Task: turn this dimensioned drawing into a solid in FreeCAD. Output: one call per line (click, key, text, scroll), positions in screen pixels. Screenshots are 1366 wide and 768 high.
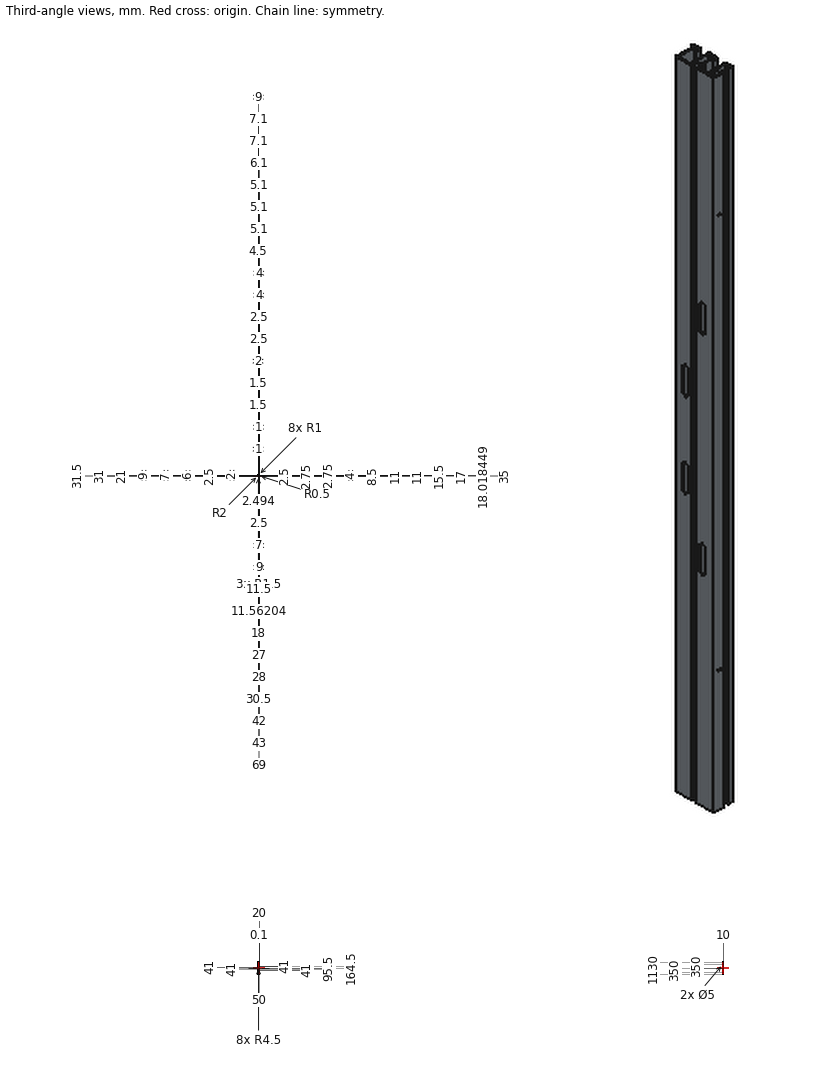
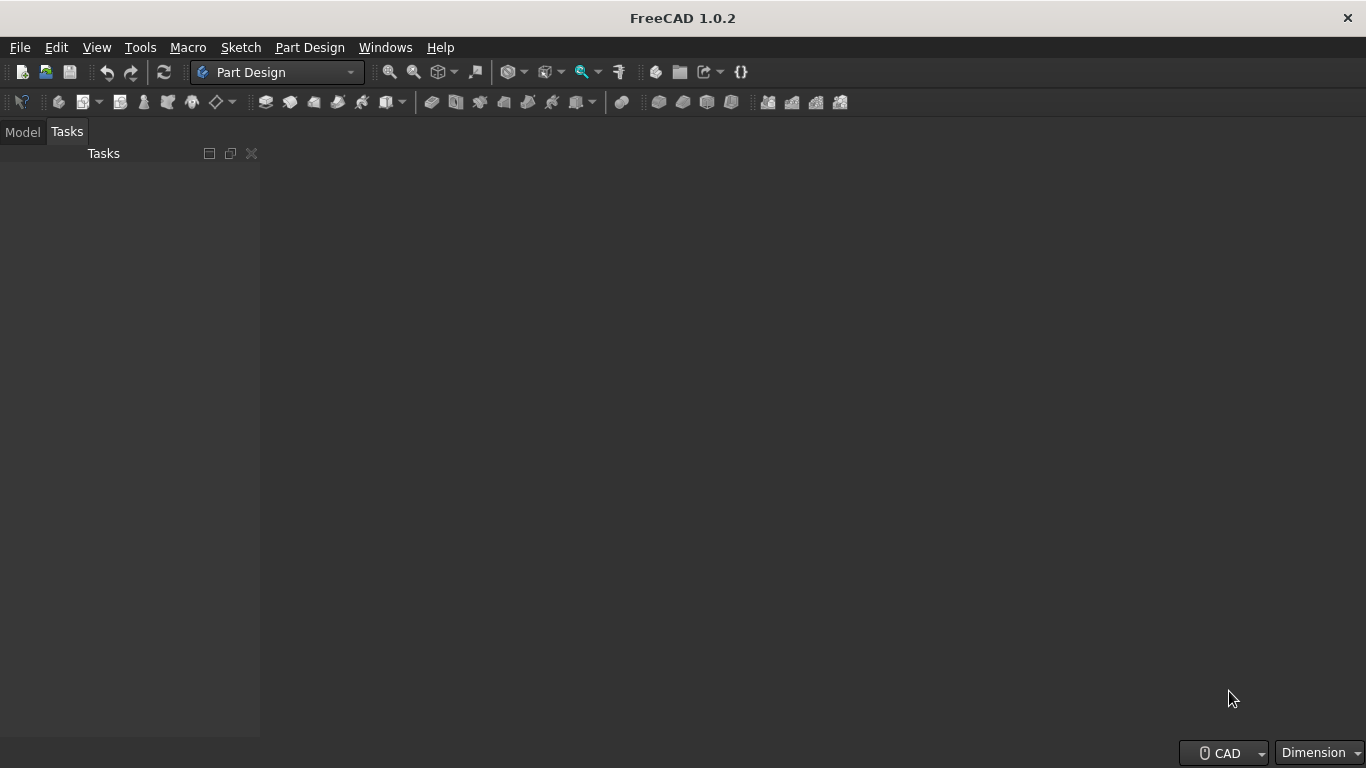
click(22, 72)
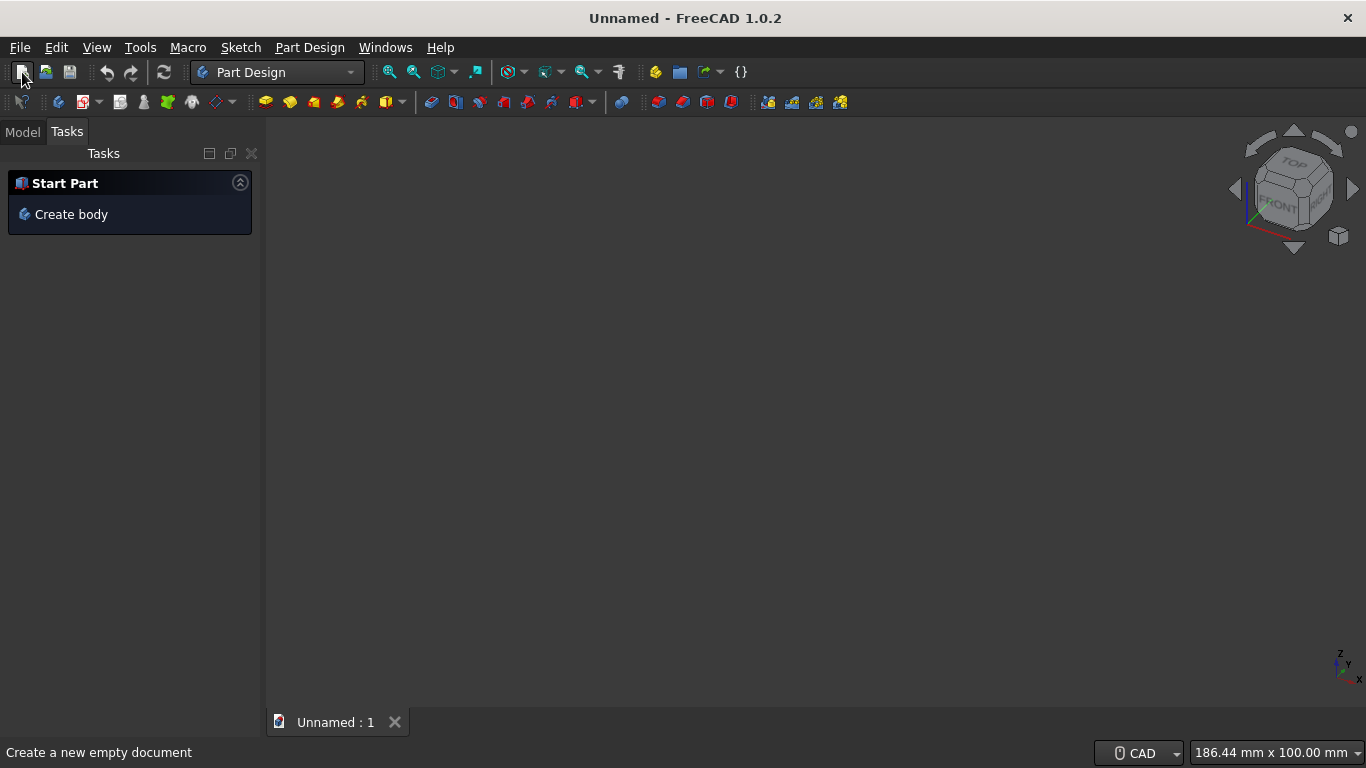
click(84, 102)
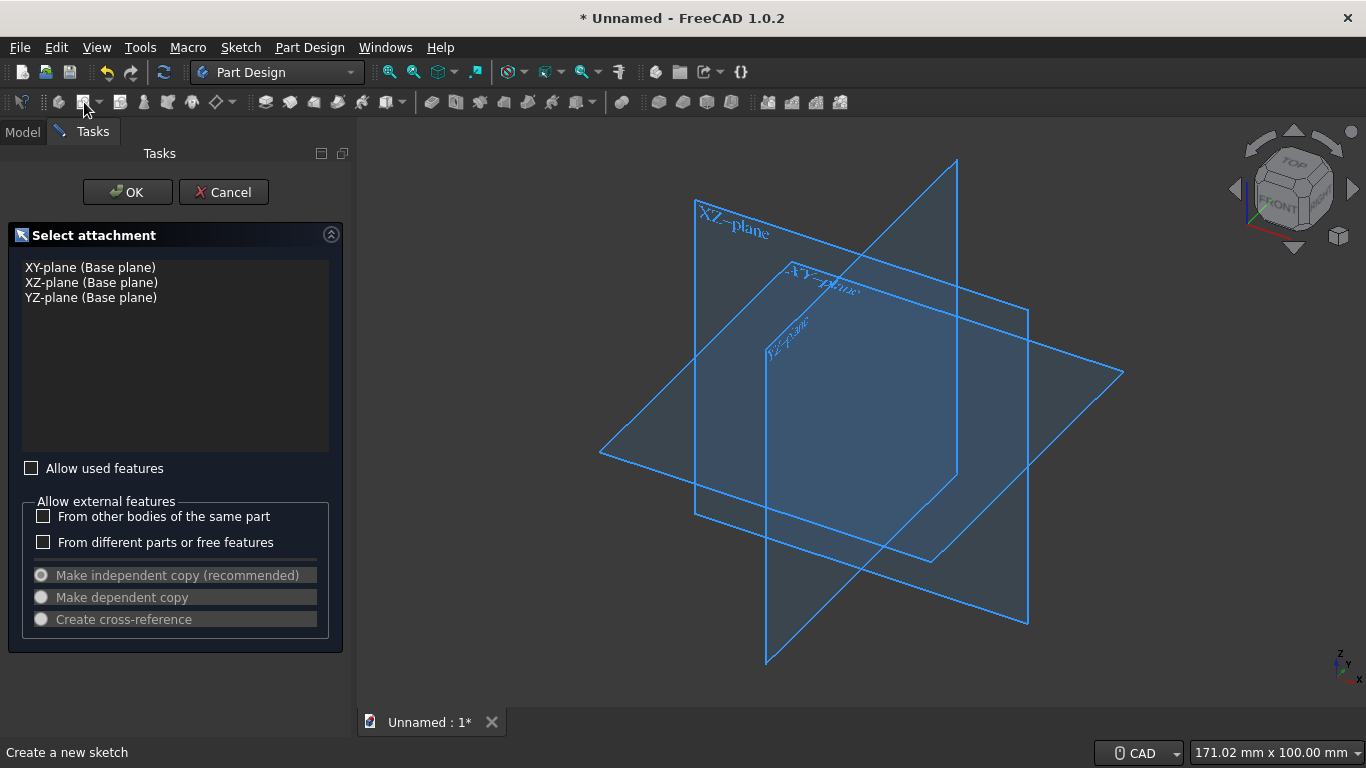
click(82, 268)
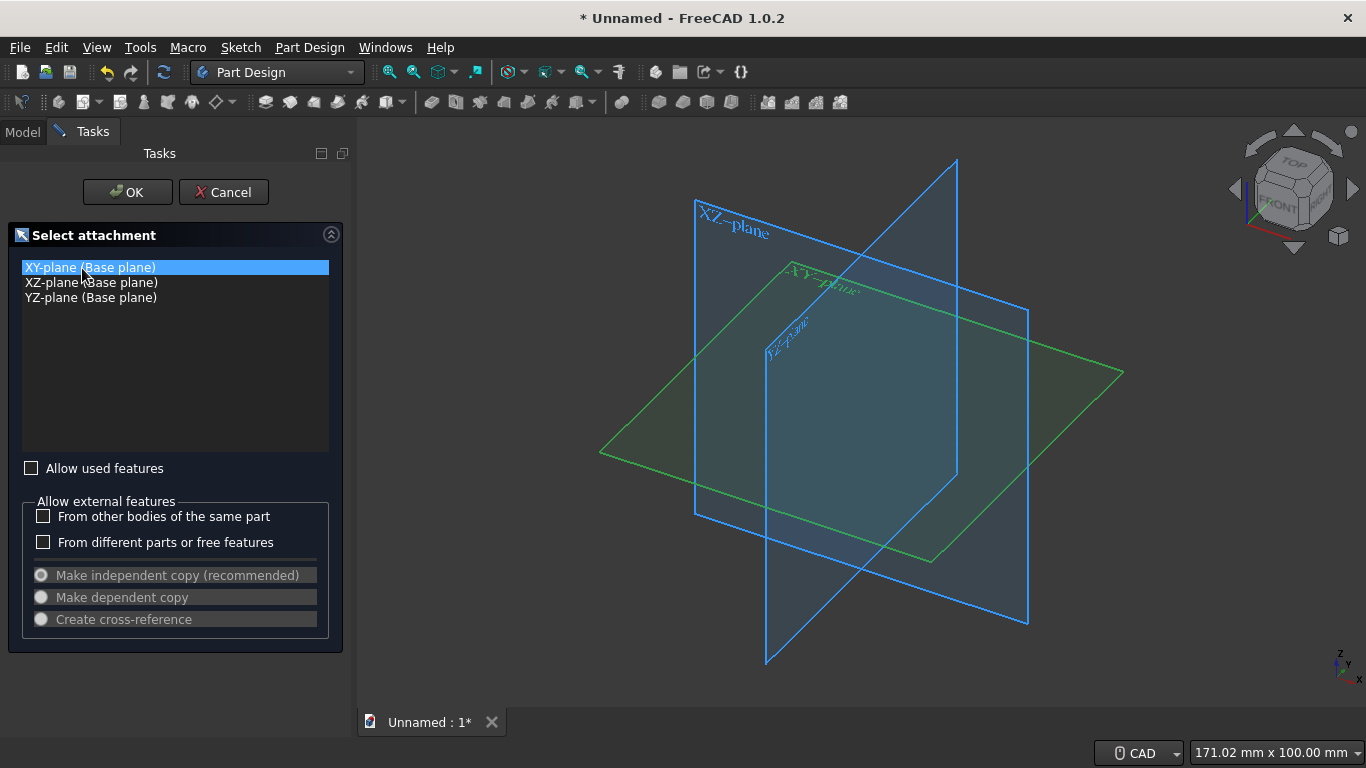
click(128, 192)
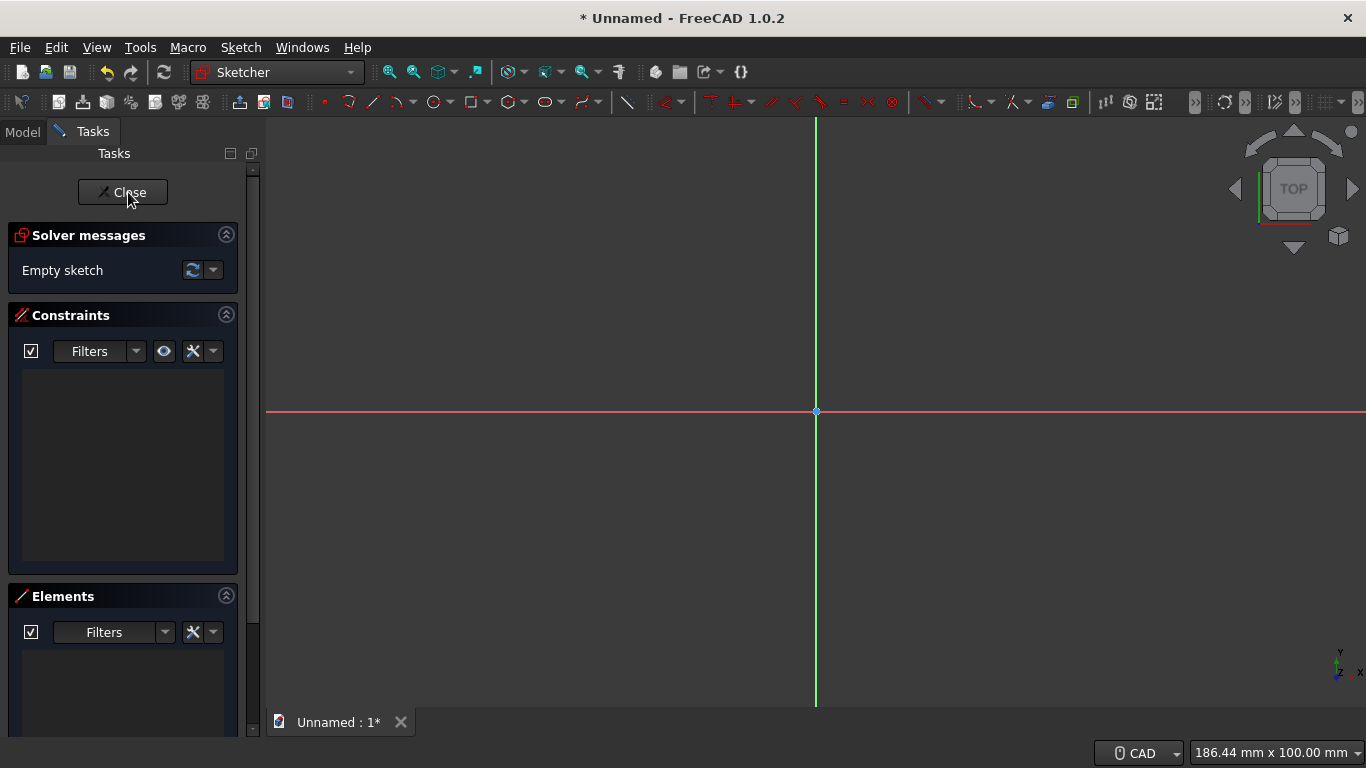
scroll(329, 145, up, 2)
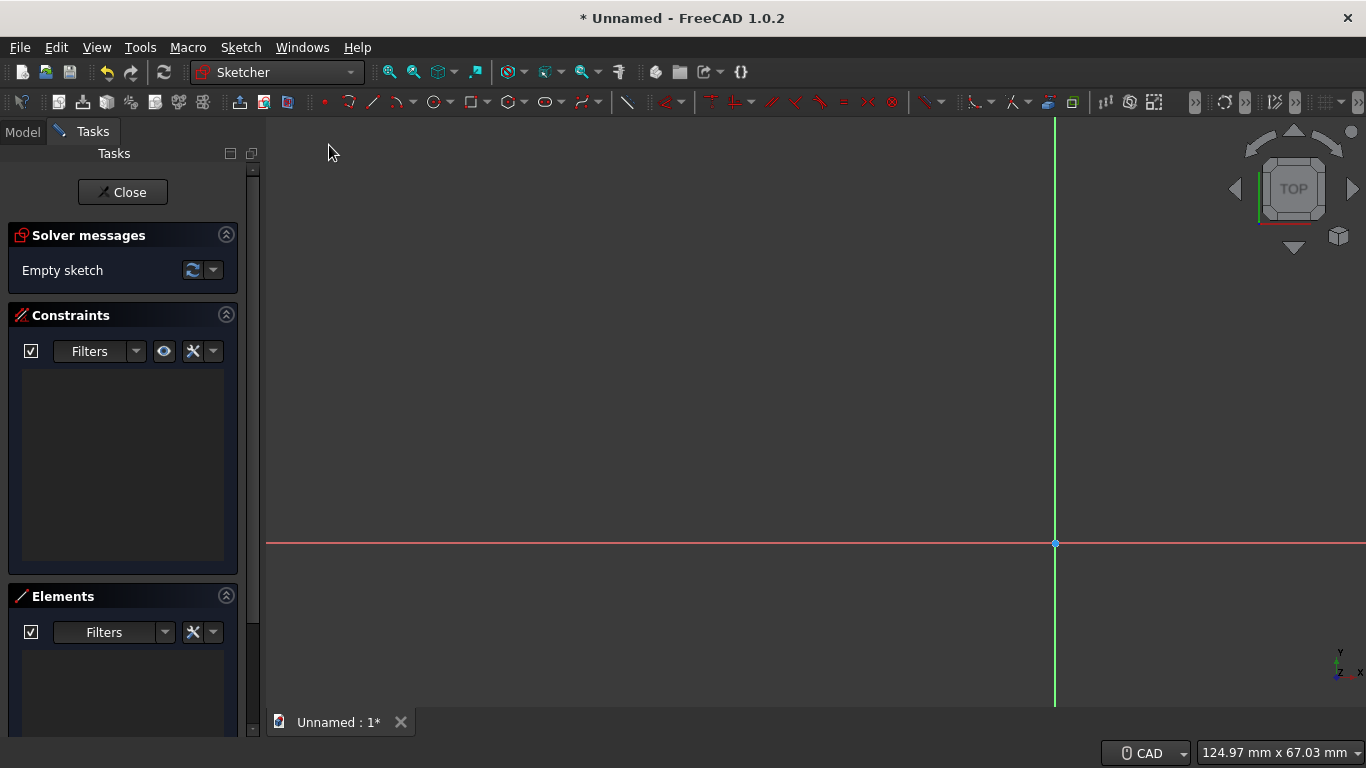
key(g)
key(l)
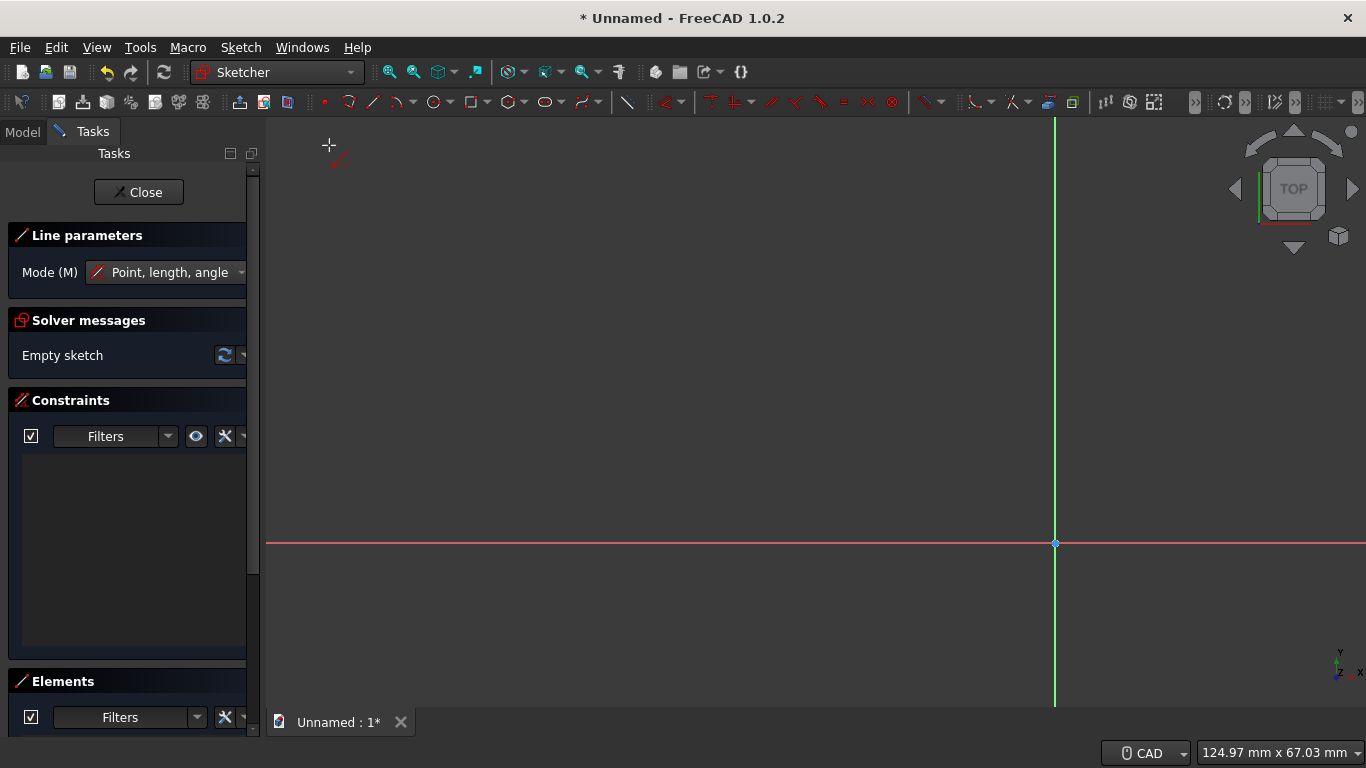
click(818, 235)
click(755, 235)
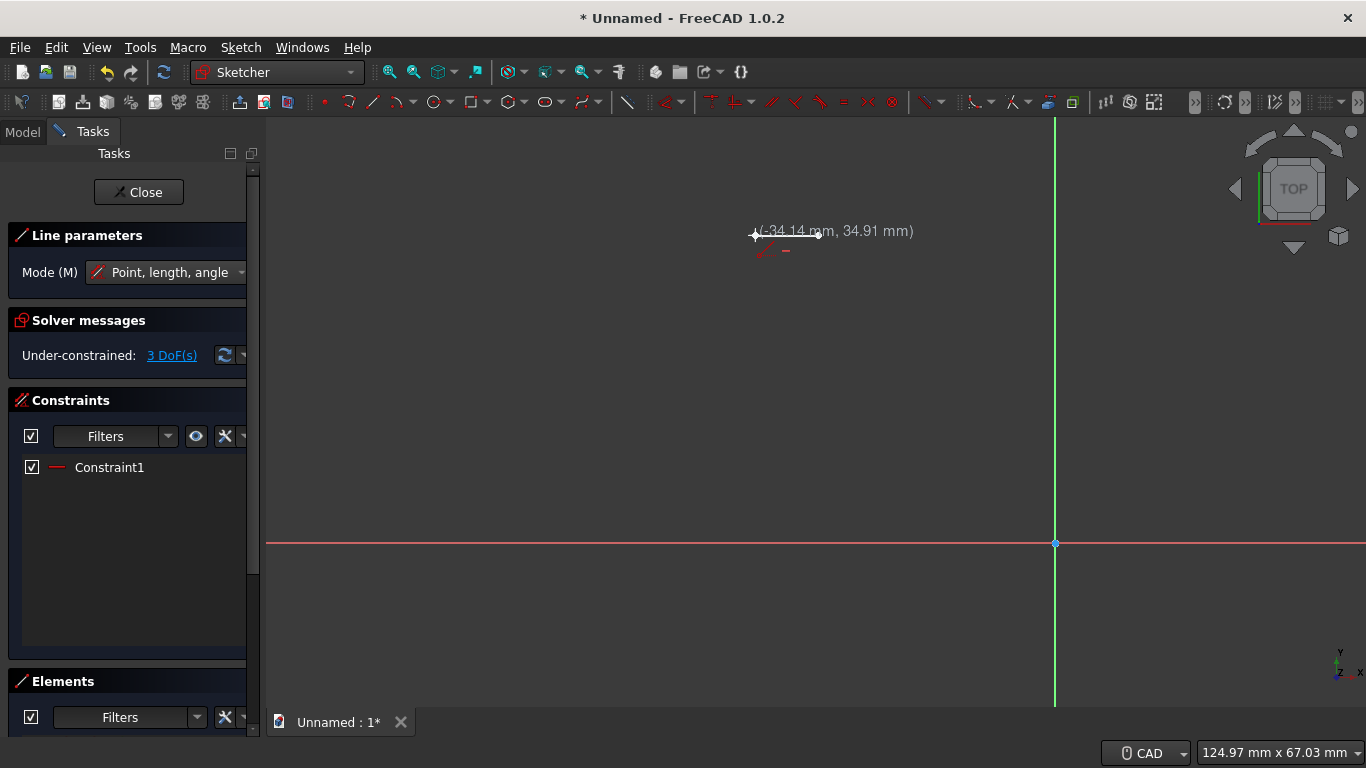
click(740, 235)
click(677, 235)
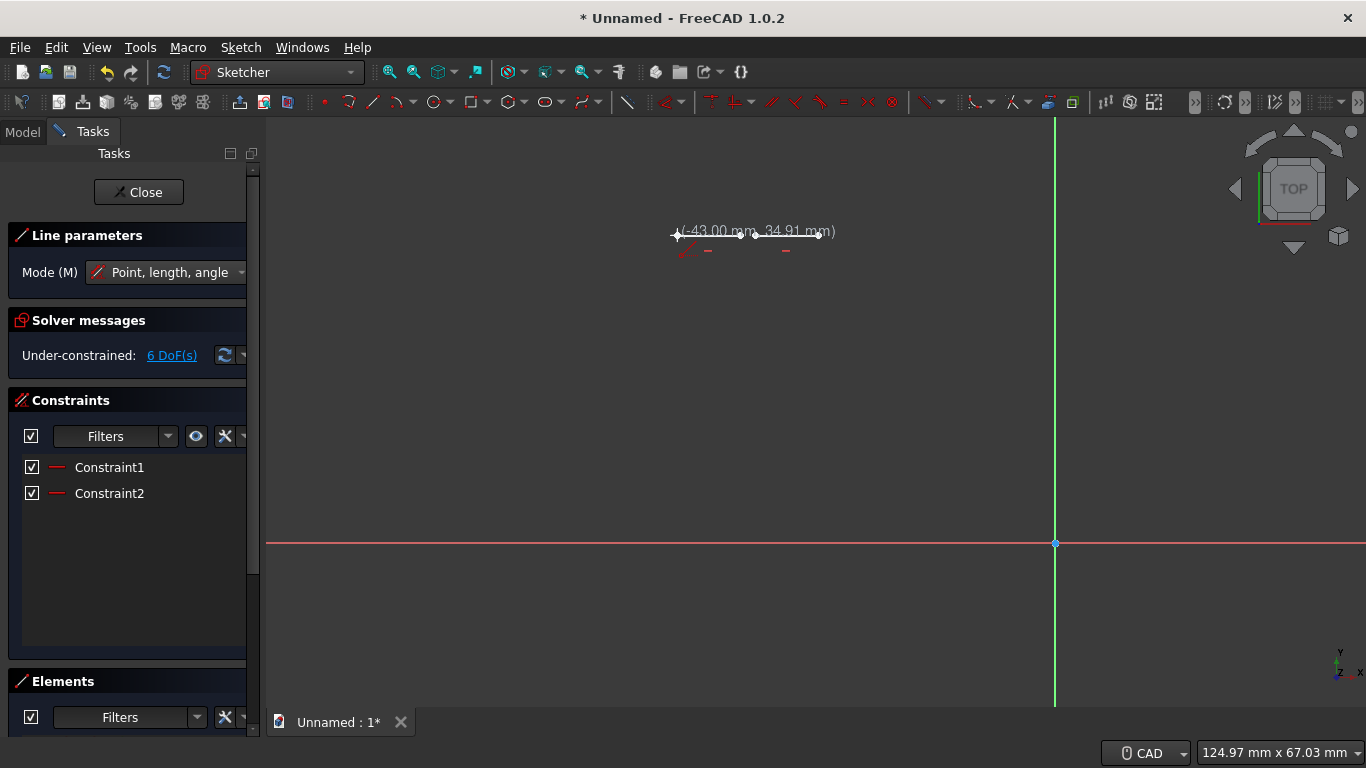
click(350, 102)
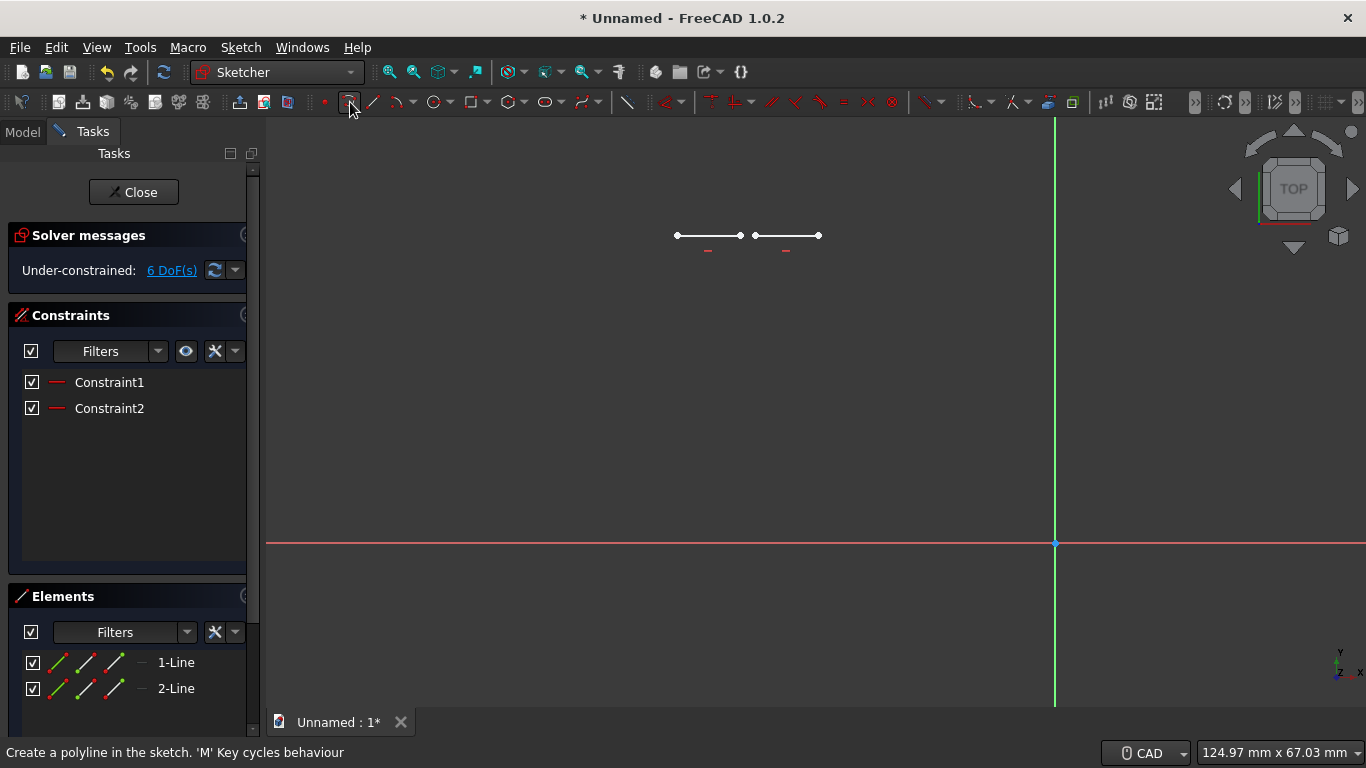
scroll(668, 244, up, 2)